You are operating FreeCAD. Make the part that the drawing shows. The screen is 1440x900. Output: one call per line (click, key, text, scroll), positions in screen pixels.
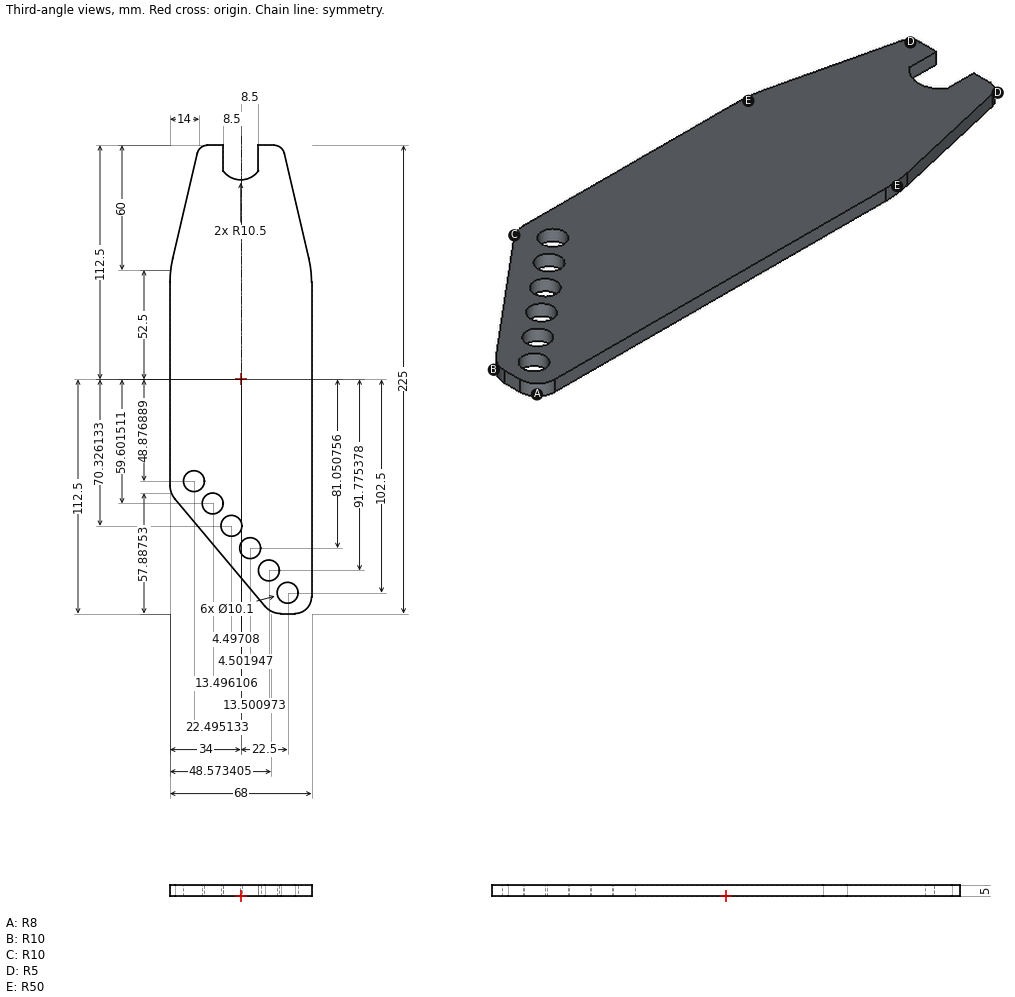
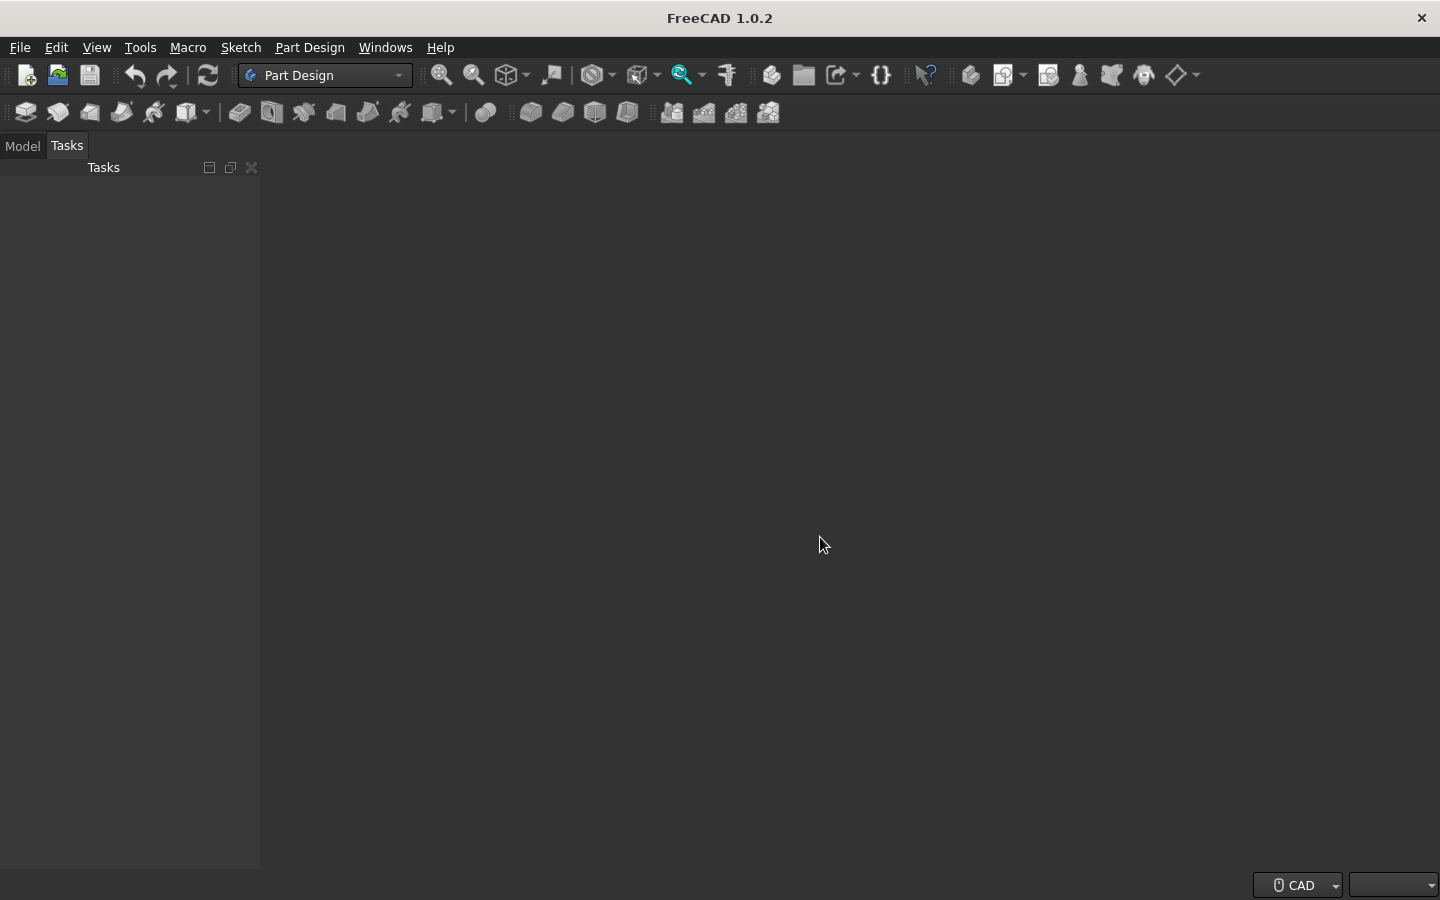
key(ctrl+n)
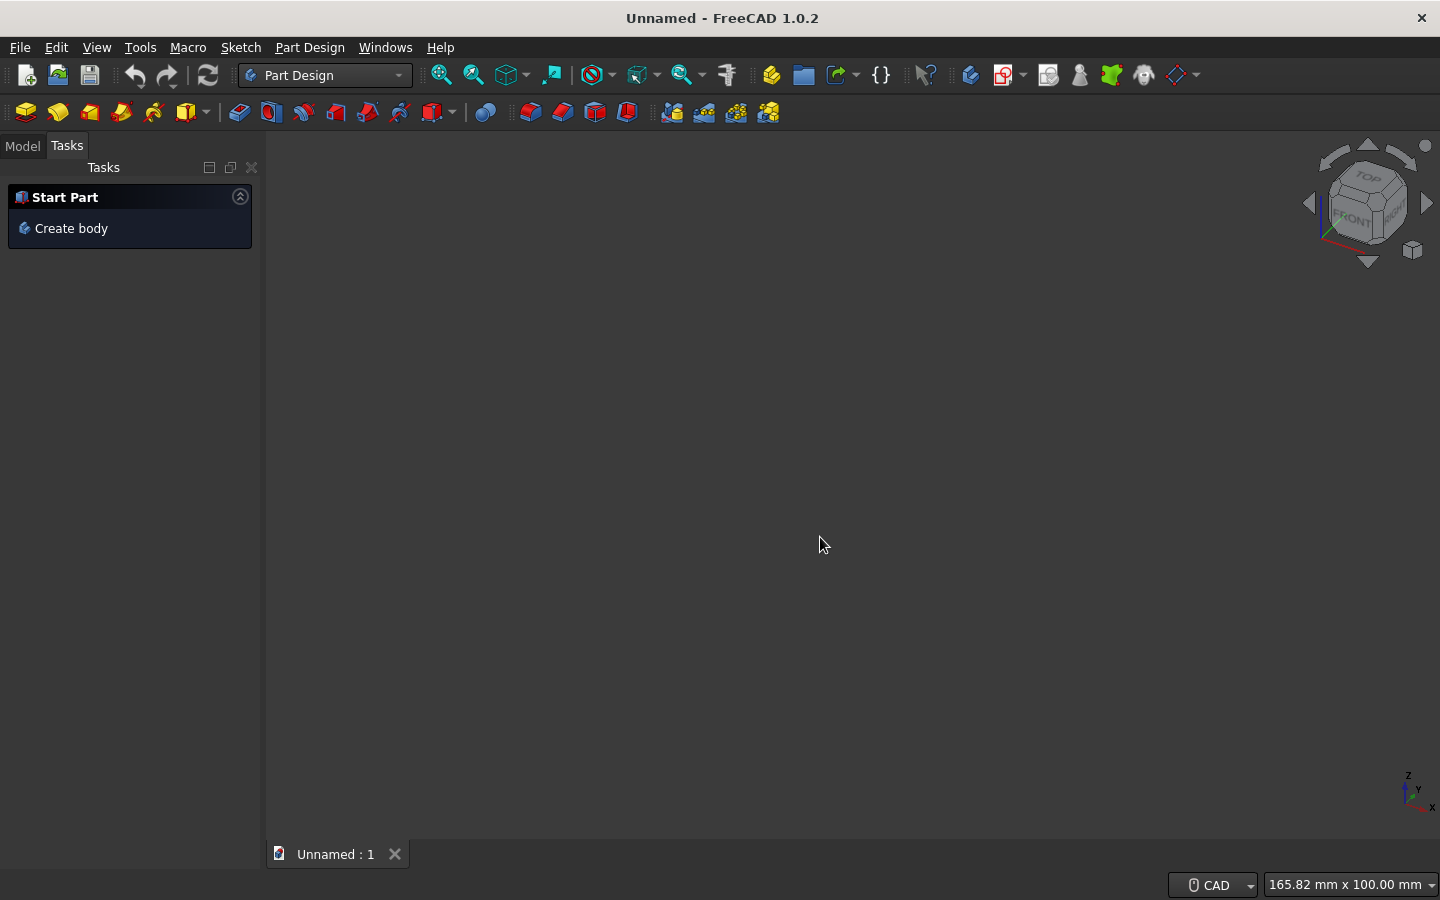
click(1004, 76)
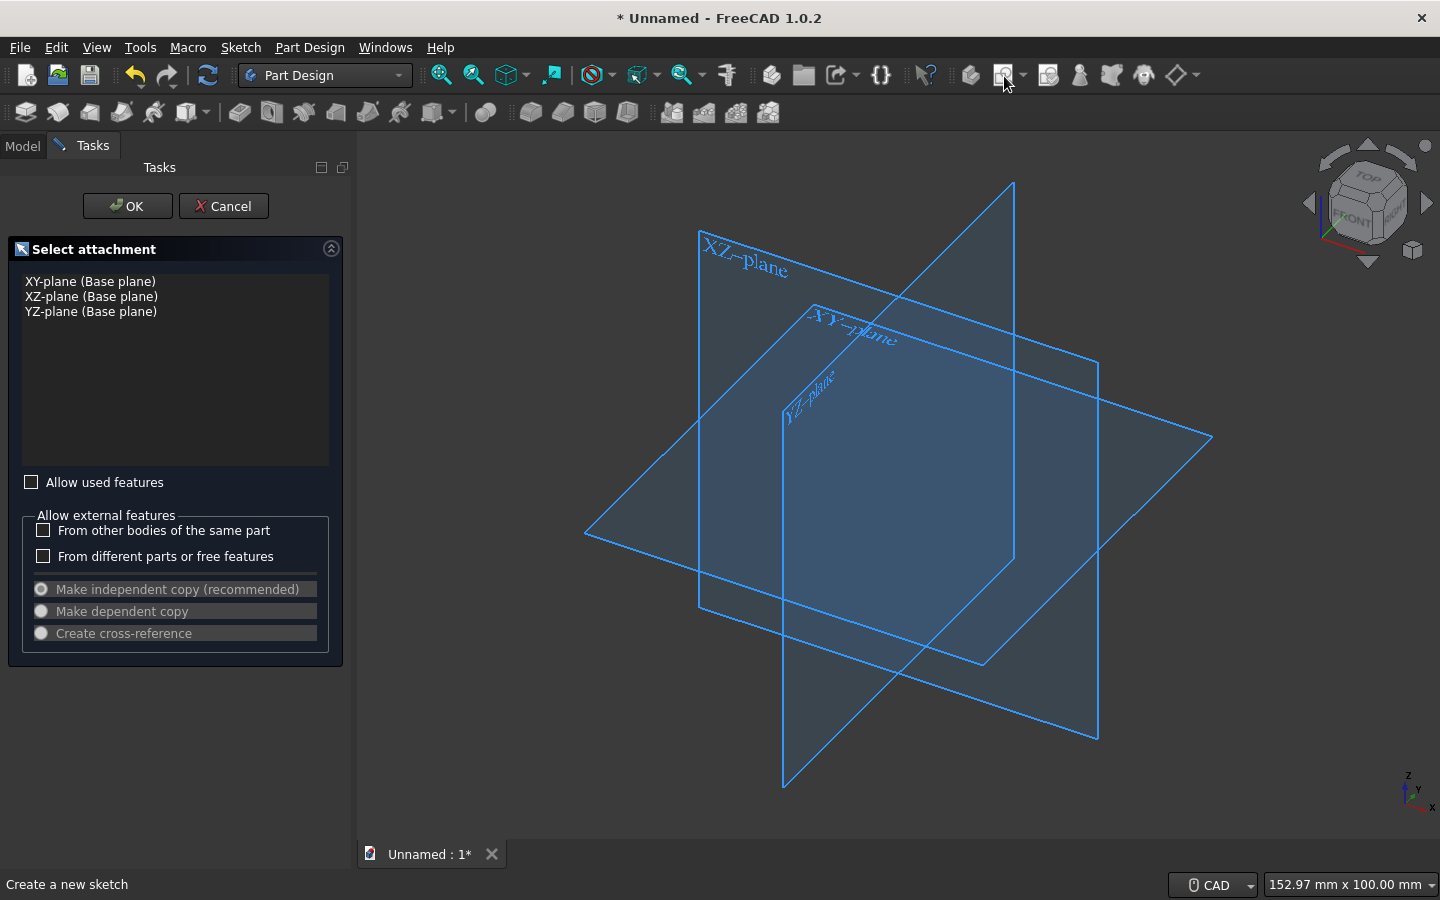
click(82, 282)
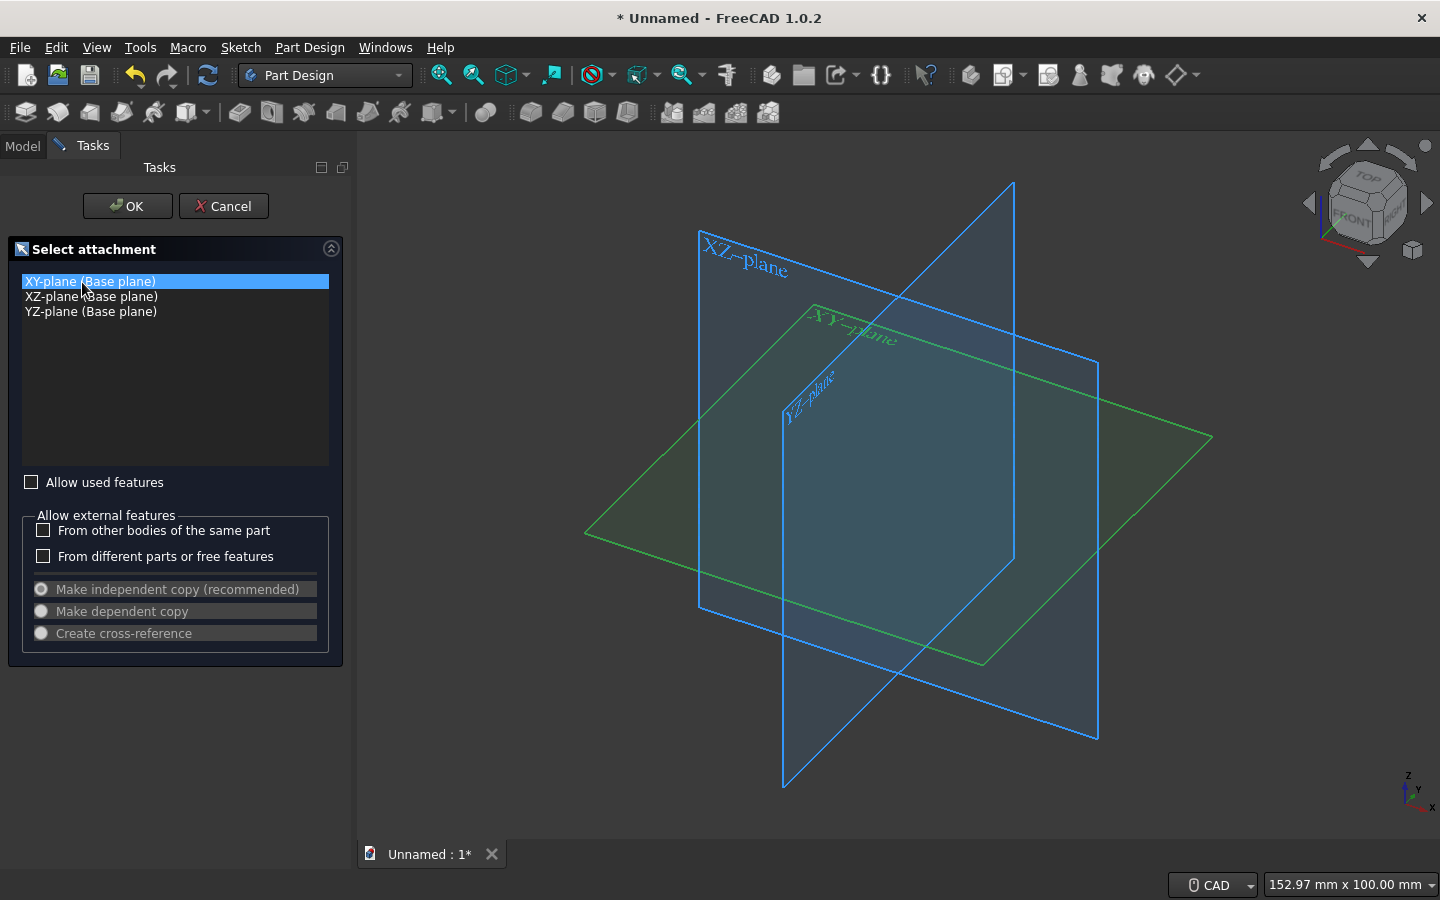
click(128, 206)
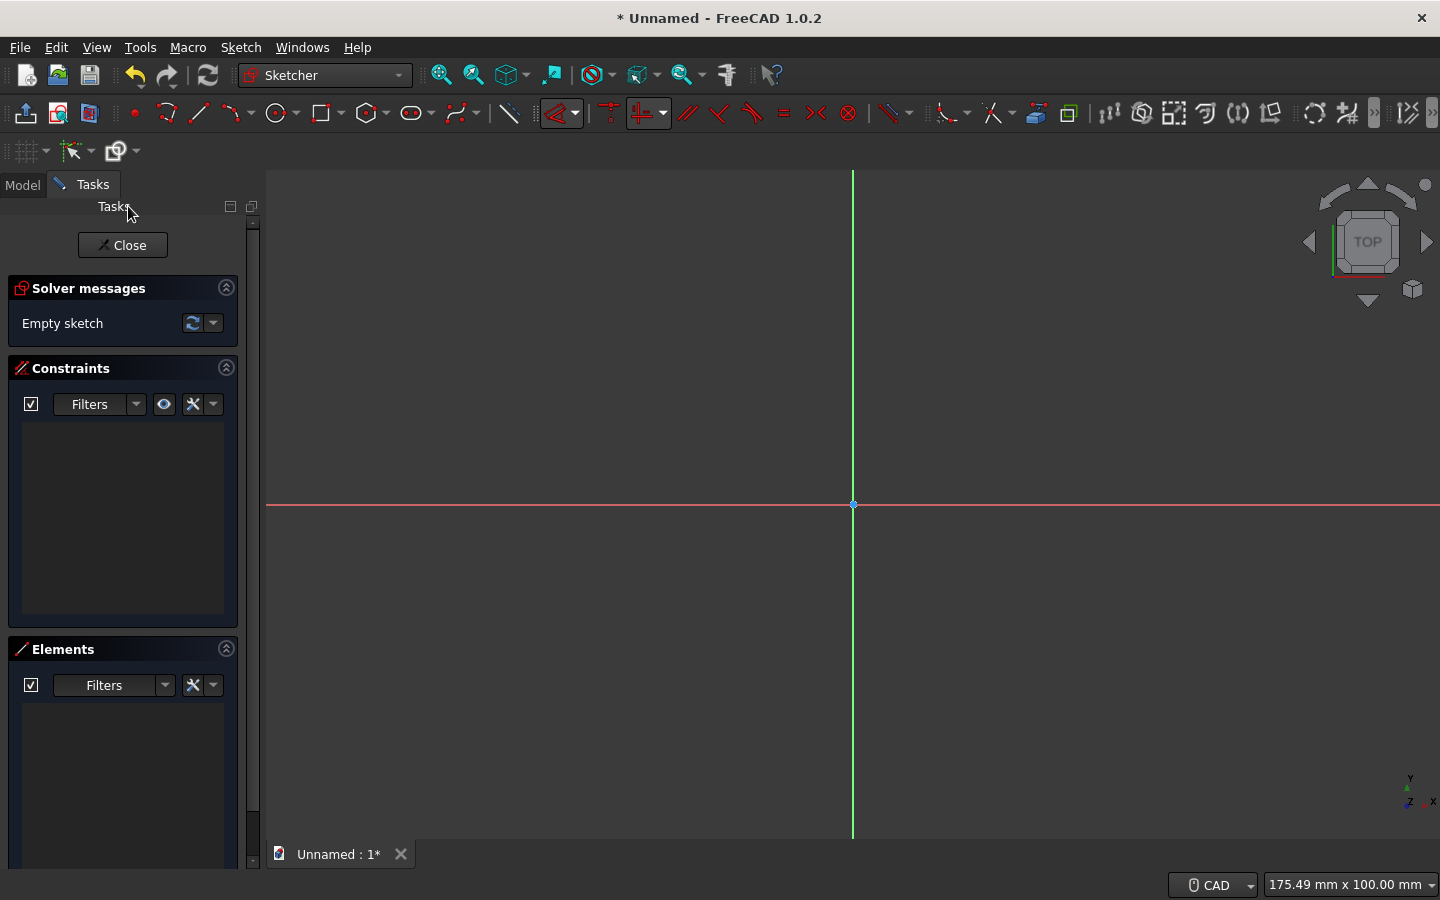
scroll(755, 504, down, 6)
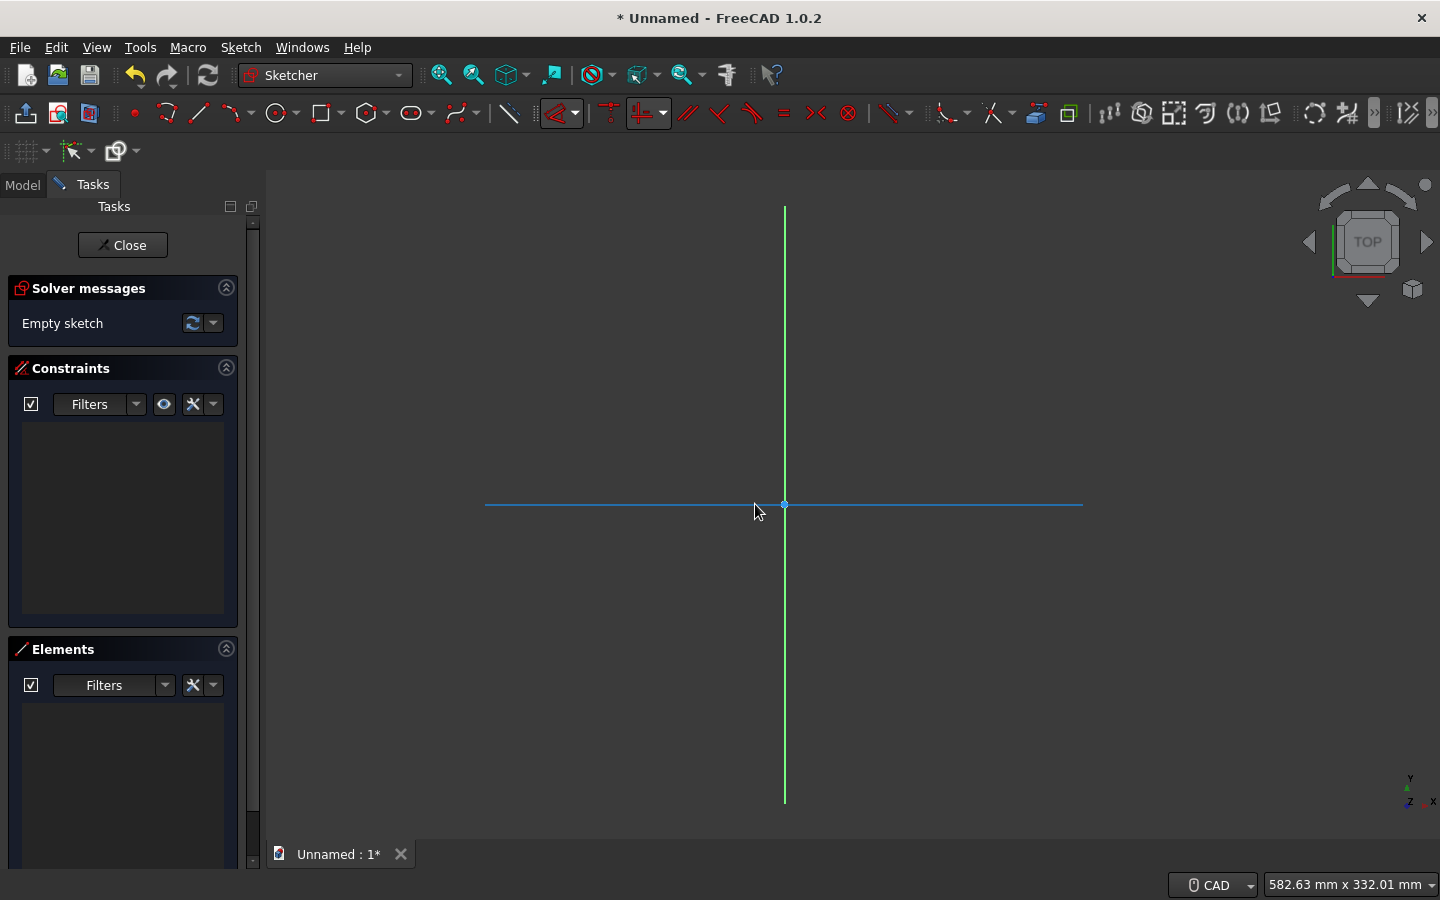
key(g)
key(v)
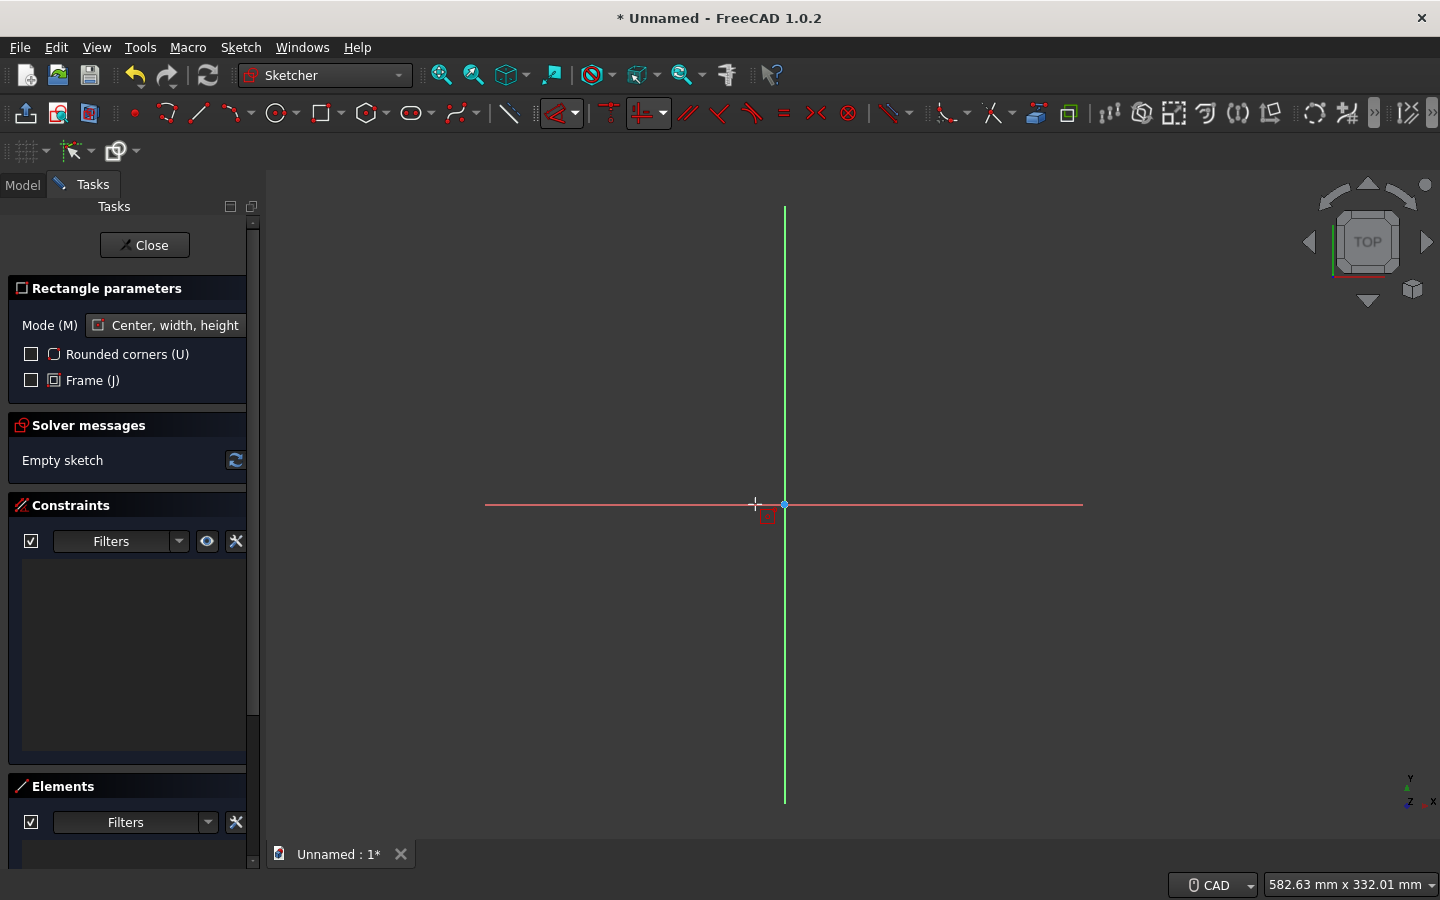
click(785, 504)
click(853, 278)
key(Escape)